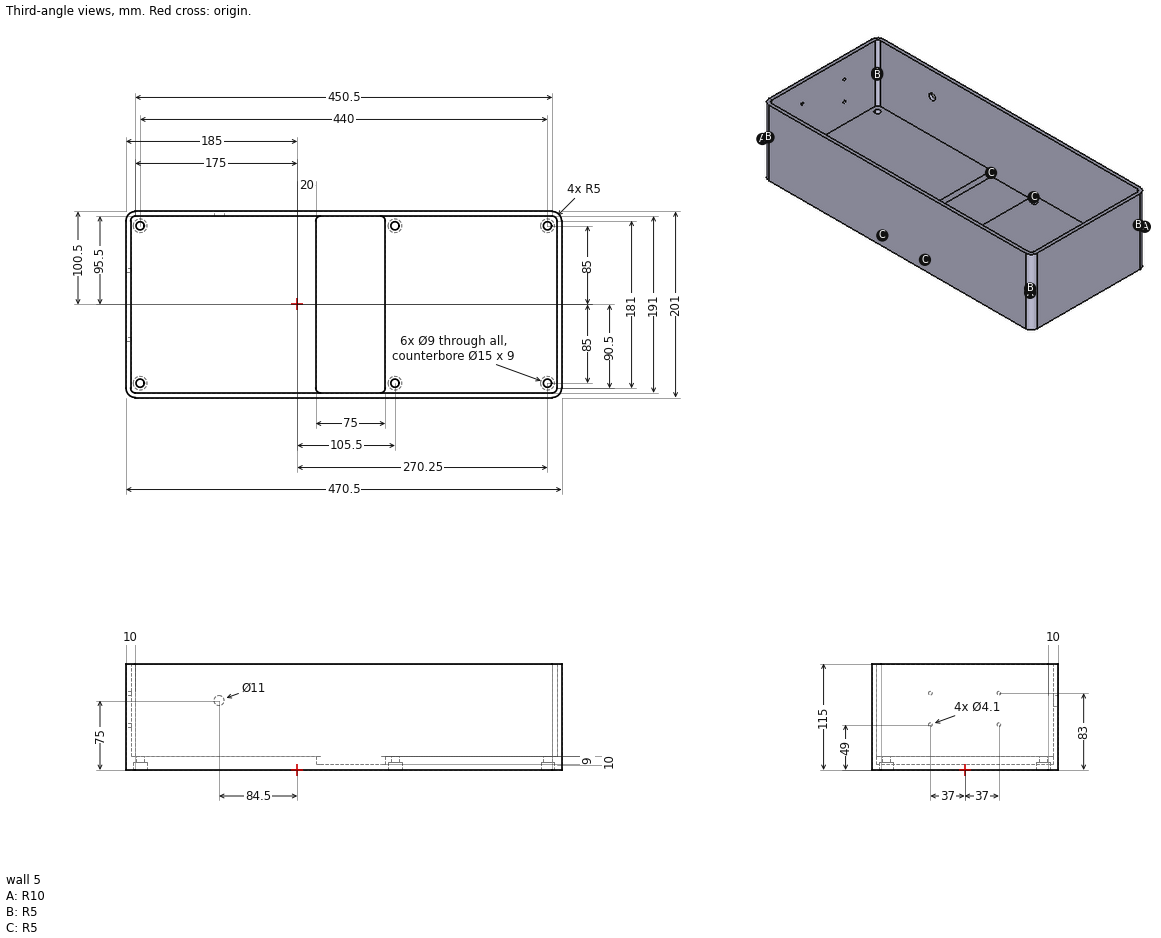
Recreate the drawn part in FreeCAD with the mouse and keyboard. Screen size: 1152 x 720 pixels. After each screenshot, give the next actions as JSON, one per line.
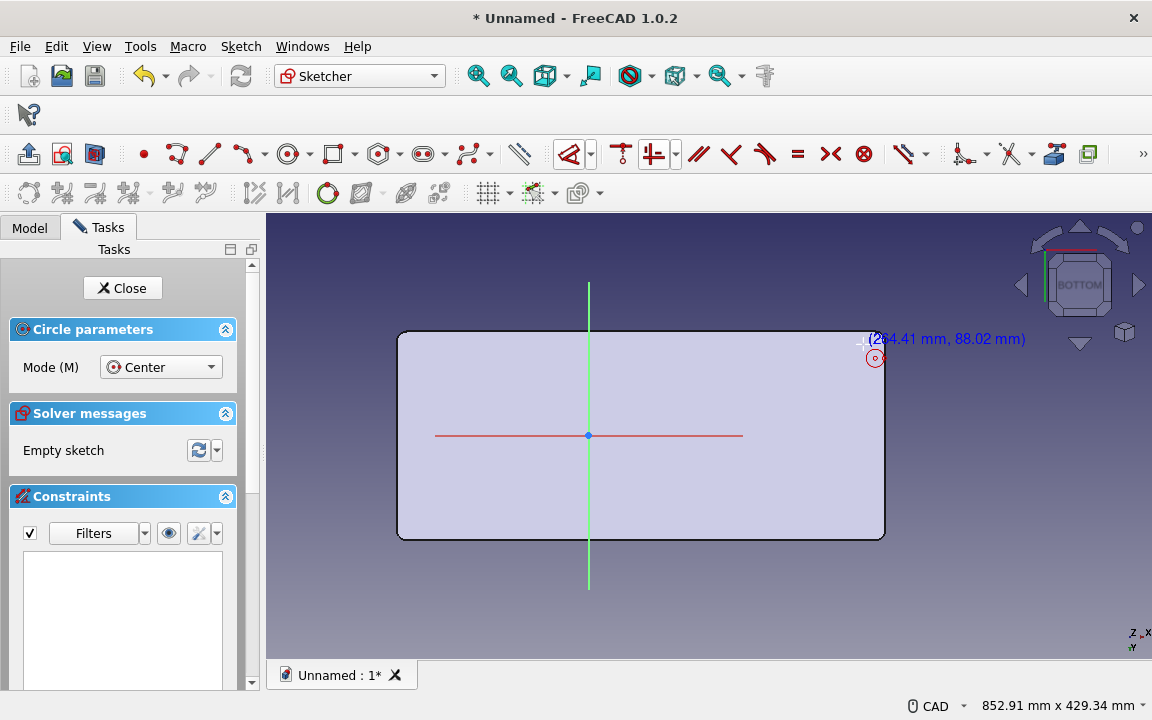
{"action": "left_click", "coordinate": [870, 348]}
{"action": "mouse_move", "coordinate": [873, 344]}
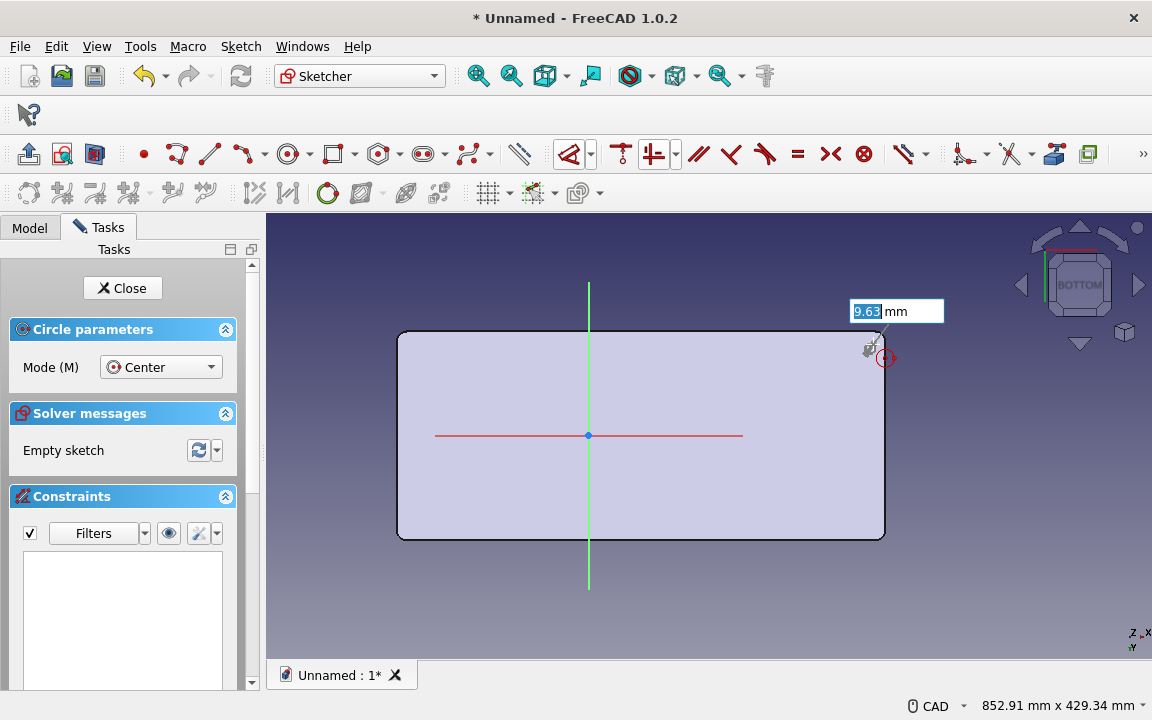
{"action": "type", "text": "9"}
{"action": "key", "text": "Return"}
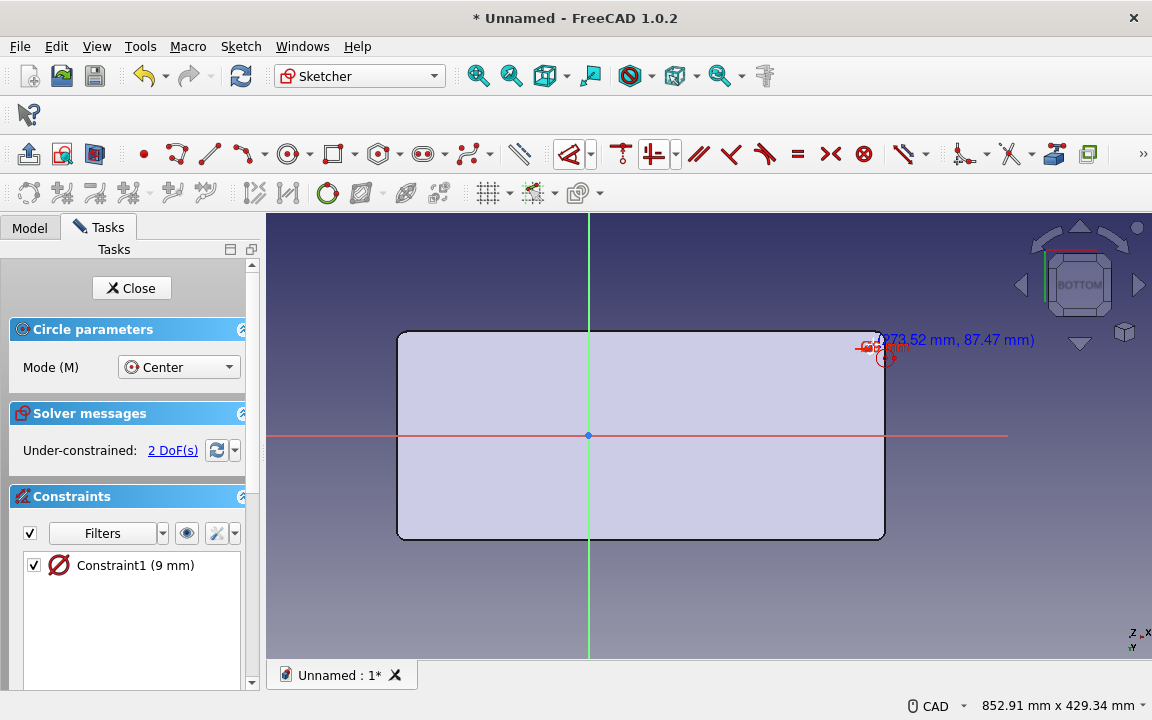
{"action": "scroll", "coordinate": [870, 524], "scroll_direction": "up", "scroll_amount": 8}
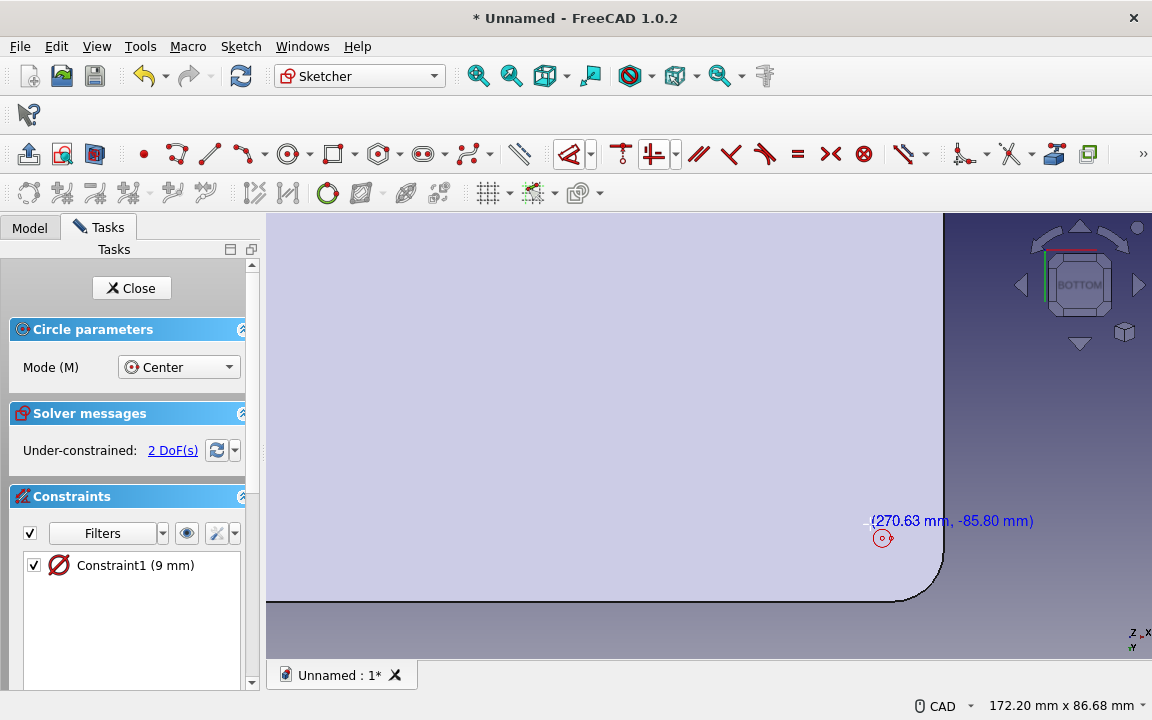
{"action": "scroll", "coordinate": [870, 525], "scroll_direction": "down", "scroll_amount": 8}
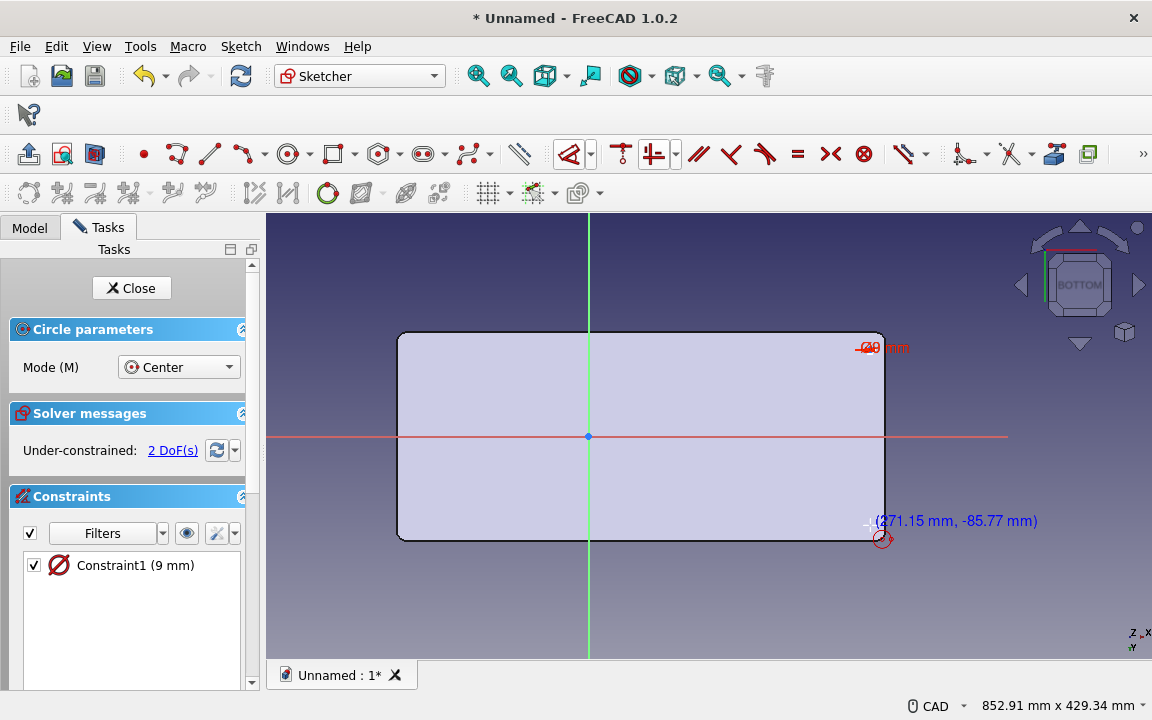
{"action": "left_click", "coordinate": [870, 525]}
{"action": "mouse_move", "coordinate": [873, 522]}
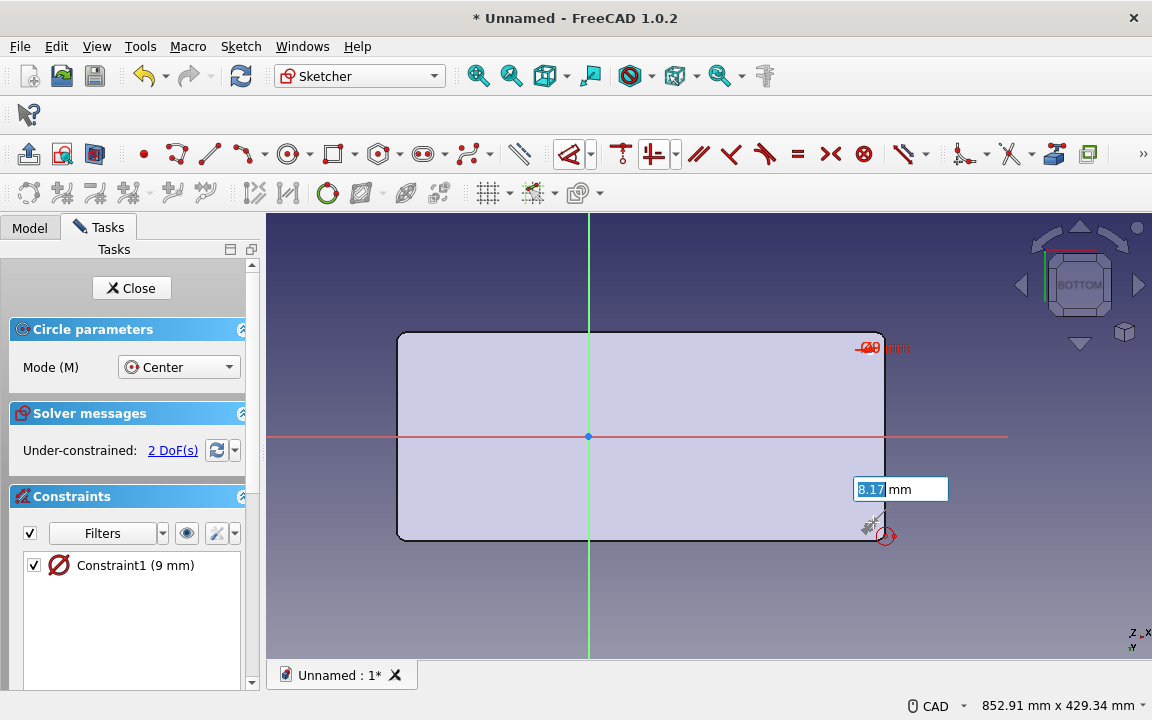
{"action": "type", "text": "9"}
{"action": "key", "text": "Return"}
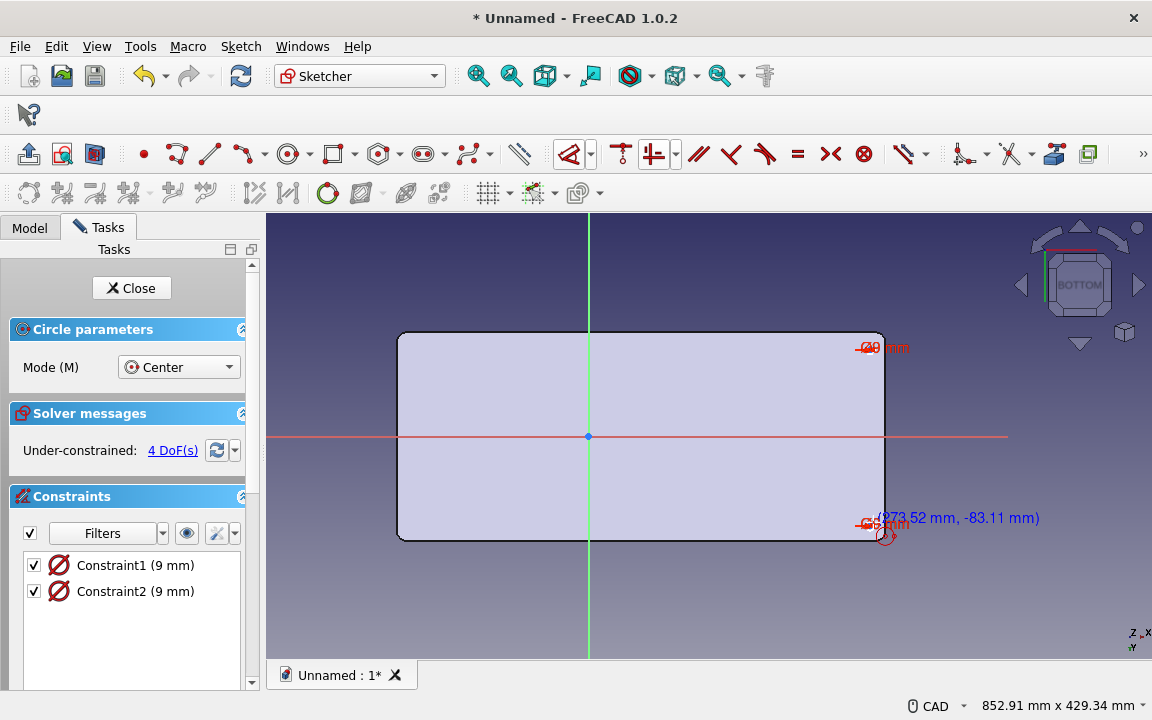
{"action": "scroll", "coordinate": [413, 525], "scroll_direction": "up", "scroll_amount": 8}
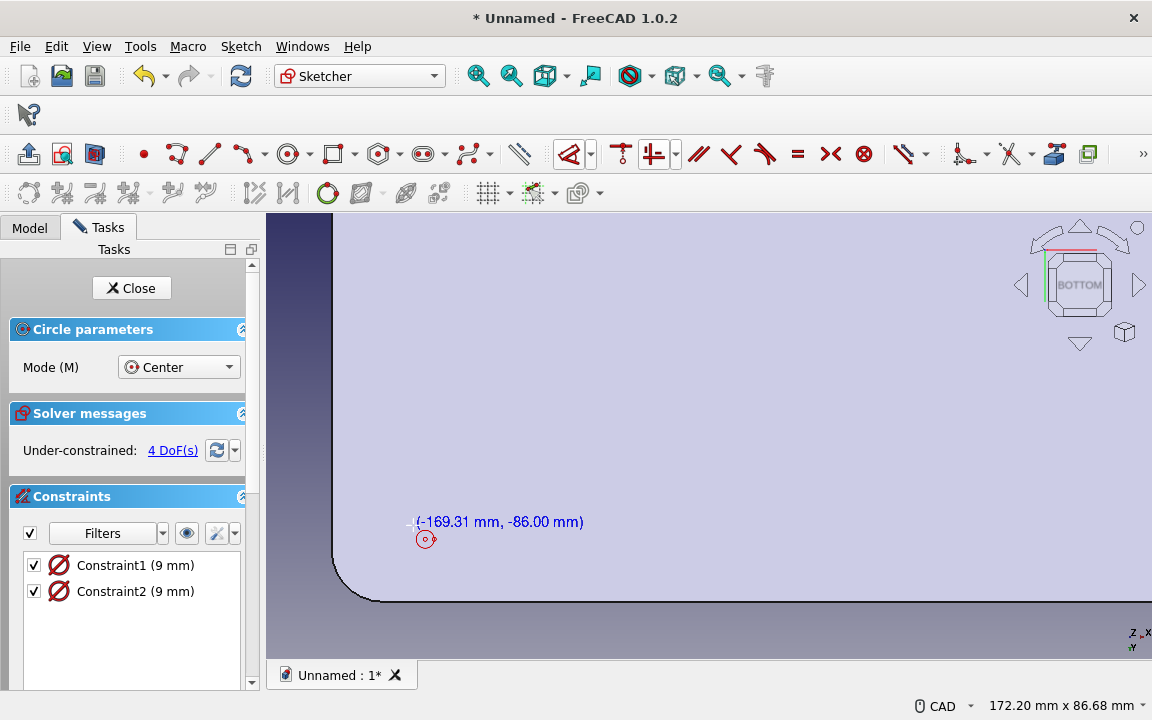
{"action": "scroll", "coordinate": [412, 525], "scroll_direction": "down", "scroll_amount": 8}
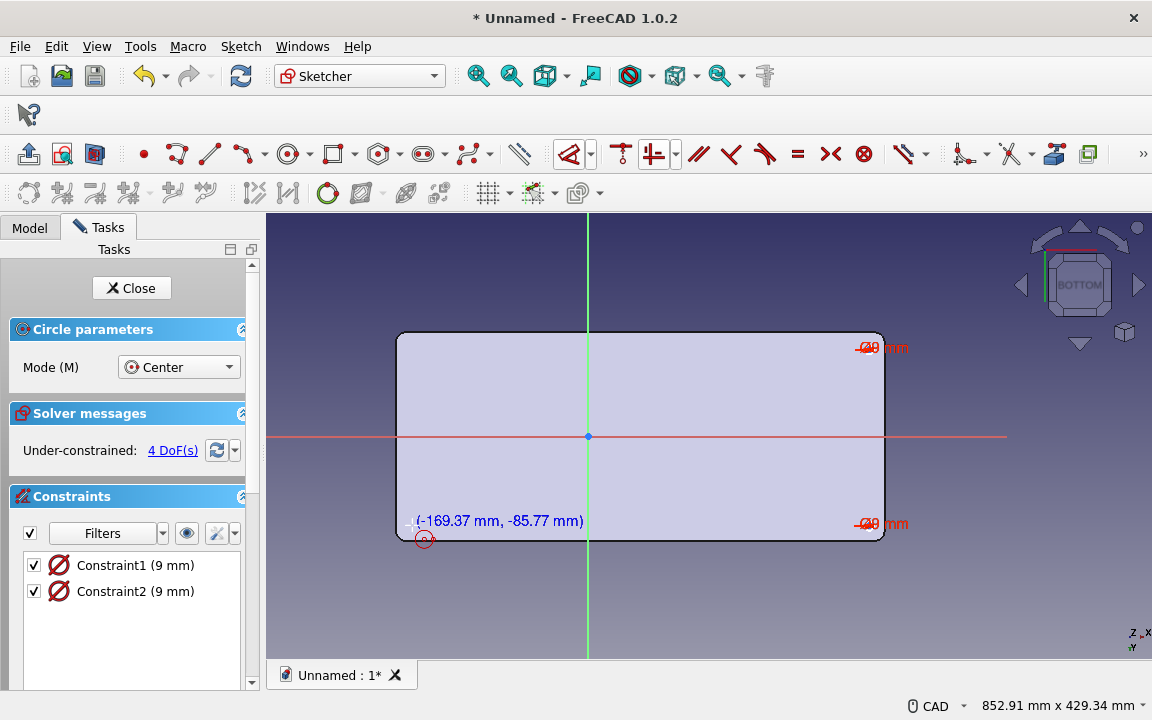
{"action": "left_click", "coordinate": [412, 525]}
{"action": "mouse_move", "coordinate": [415, 522]}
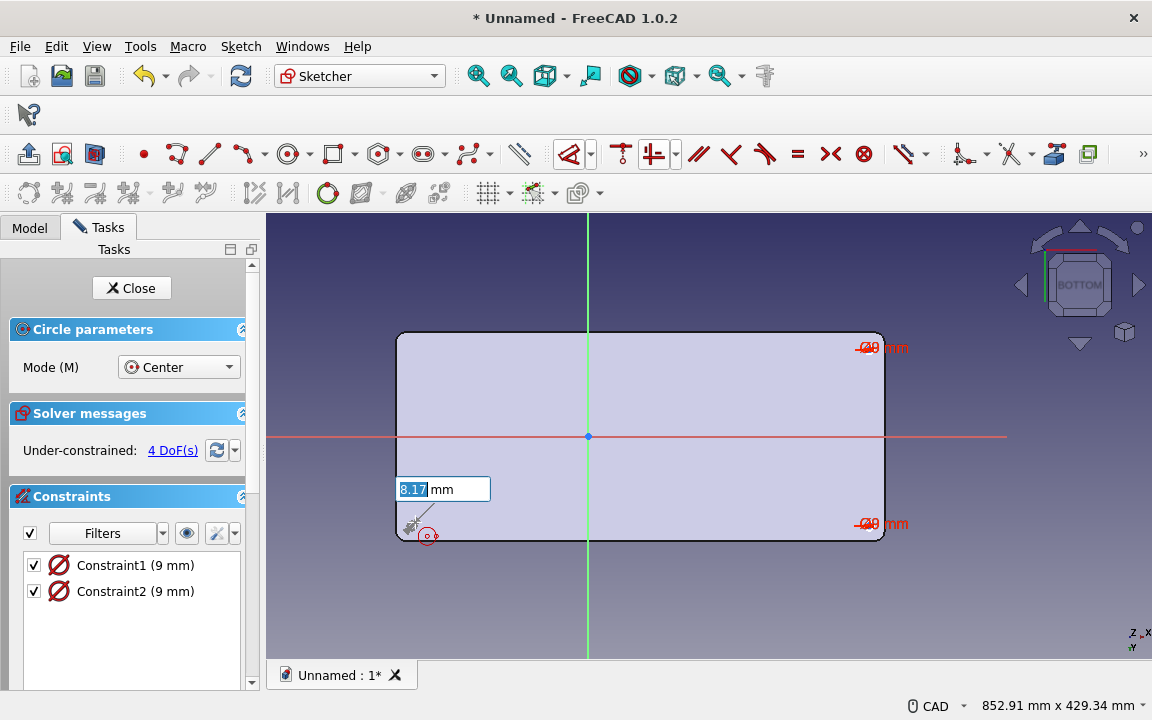
{"action": "type", "text": "9"}
{"action": "key", "text": "Return"}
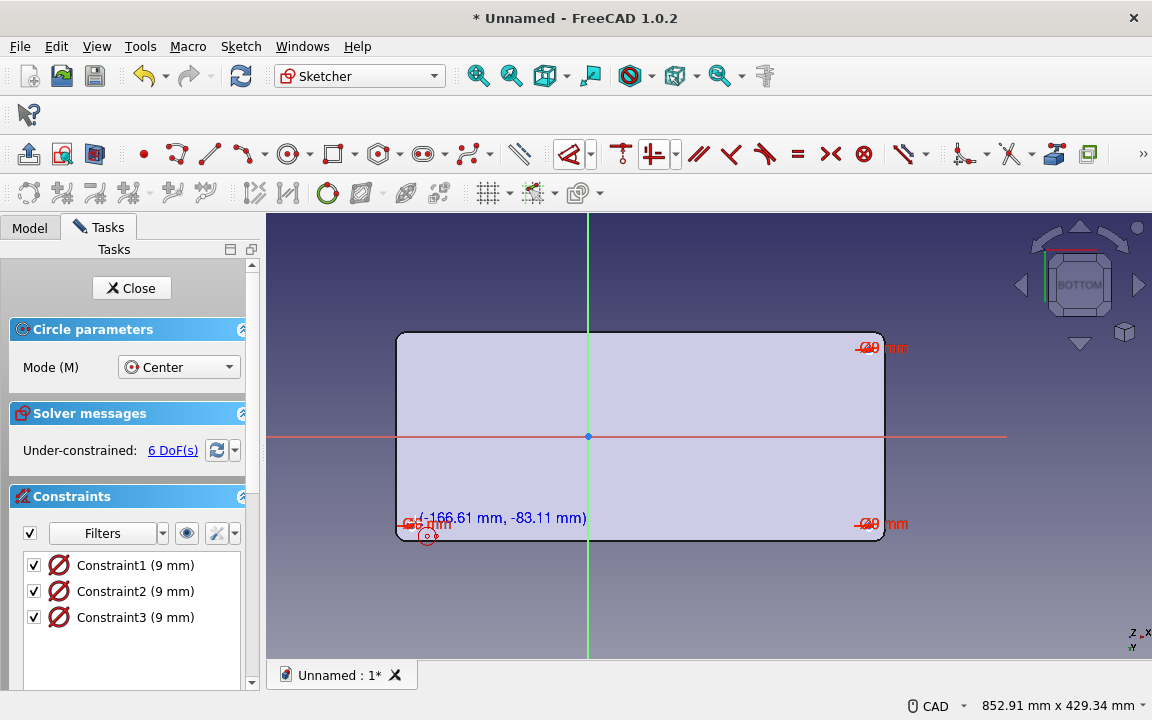
{"action": "scroll", "coordinate": [412, 348], "scroll_direction": "up", "scroll_amount": 8}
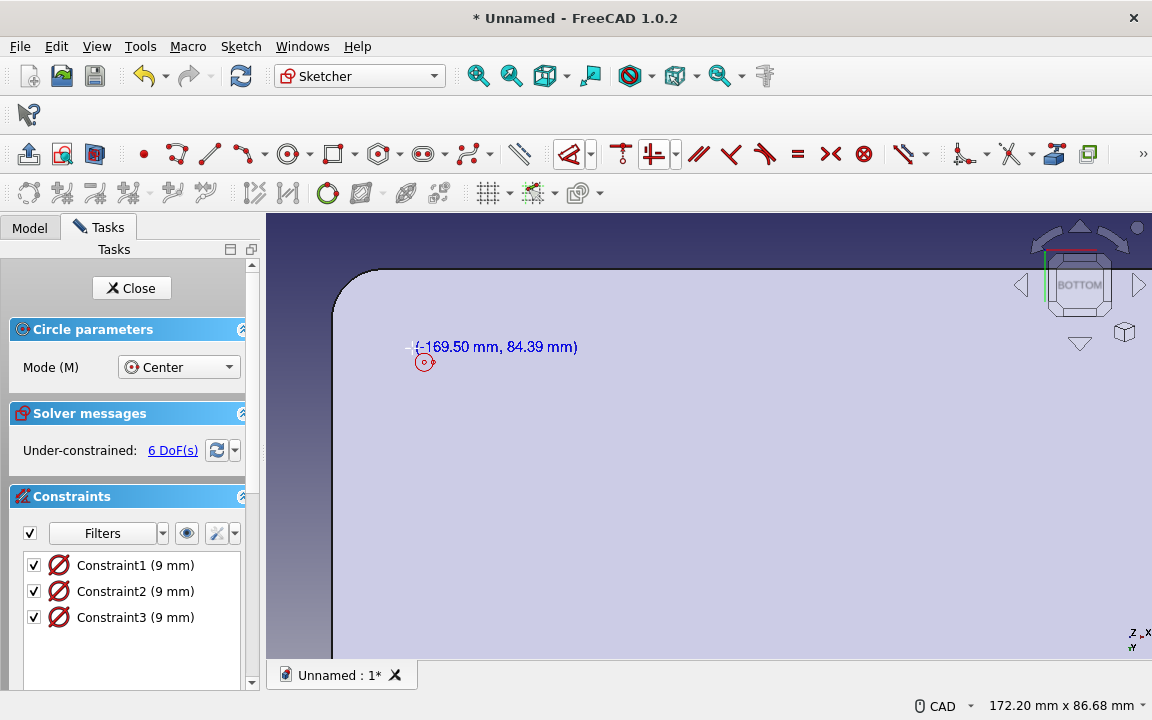
{"action": "scroll", "coordinate": [412, 347], "scroll_direction": "down", "scroll_amount": 8}